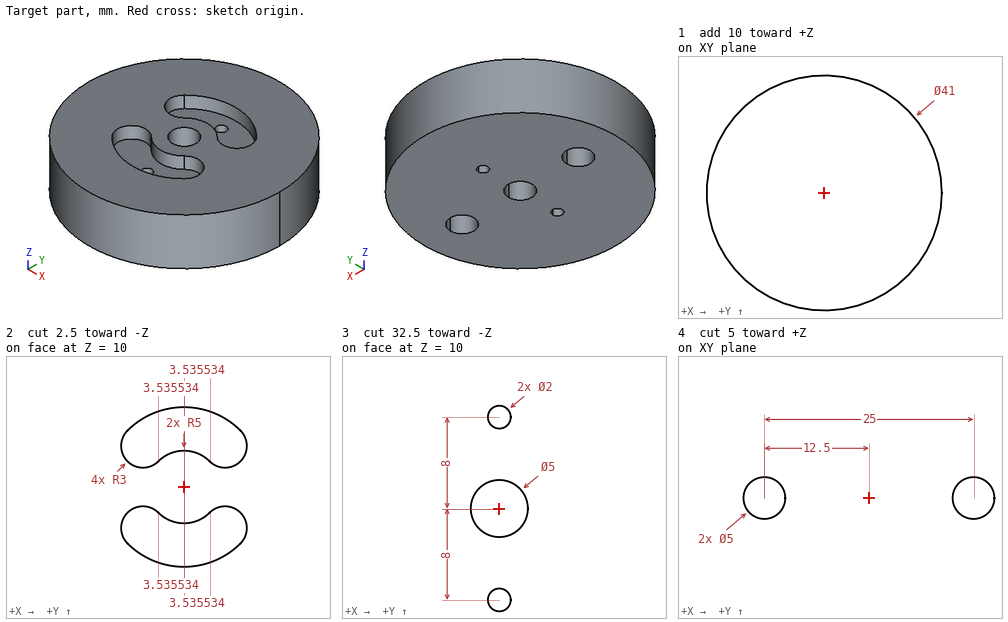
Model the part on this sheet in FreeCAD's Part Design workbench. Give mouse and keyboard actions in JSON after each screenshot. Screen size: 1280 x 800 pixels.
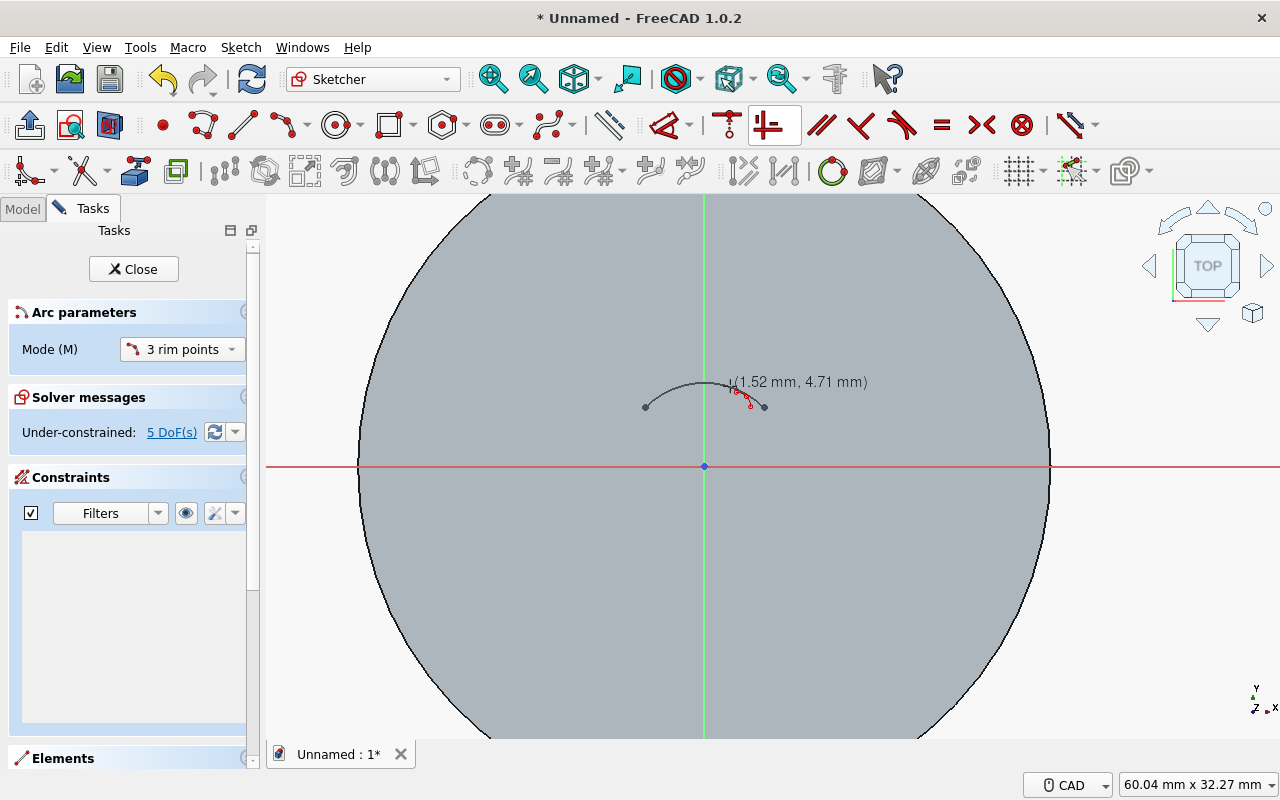
{"action": "left_click", "coordinate": [764, 408]}
{"action": "left_click", "coordinate": [836, 335]}
{"action": "left_click", "coordinate": [836, 407]}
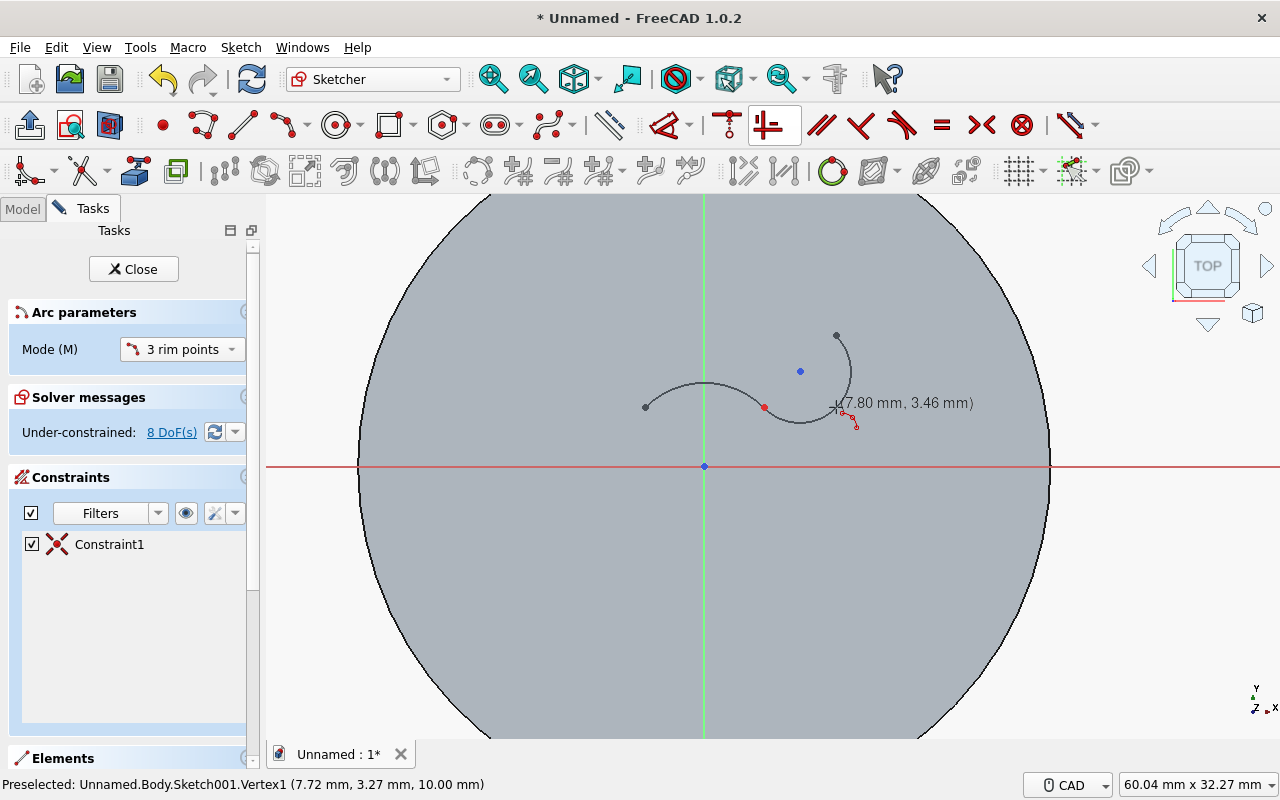
{"action": "left_click", "coordinate": [836, 336]}
{"action": "left_click", "coordinate": [573, 335]}
{"action": "left_click", "coordinate": [733, 283]}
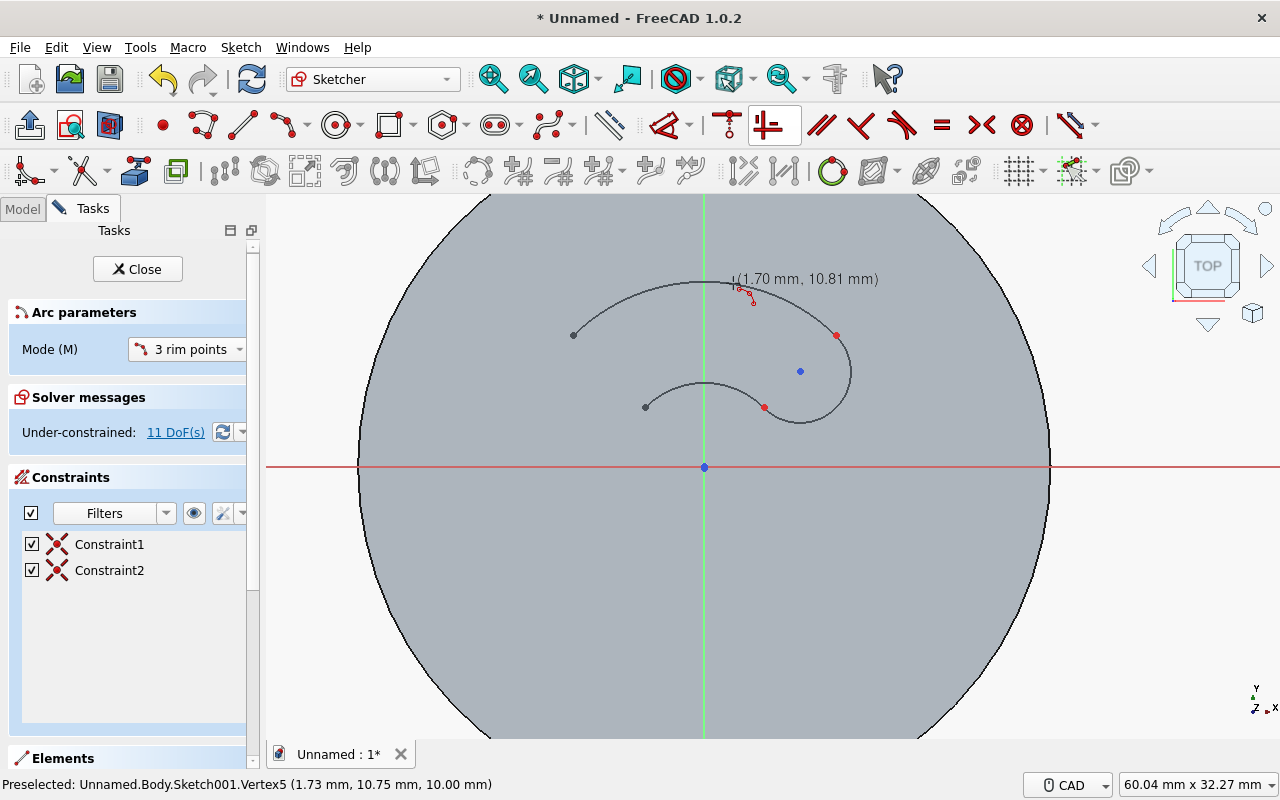
{"action": "left_click", "coordinate": [573, 336]}
{"action": "left_click", "coordinate": [645, 408]}
{"action": "left_click", "coordinate": [573, 407]}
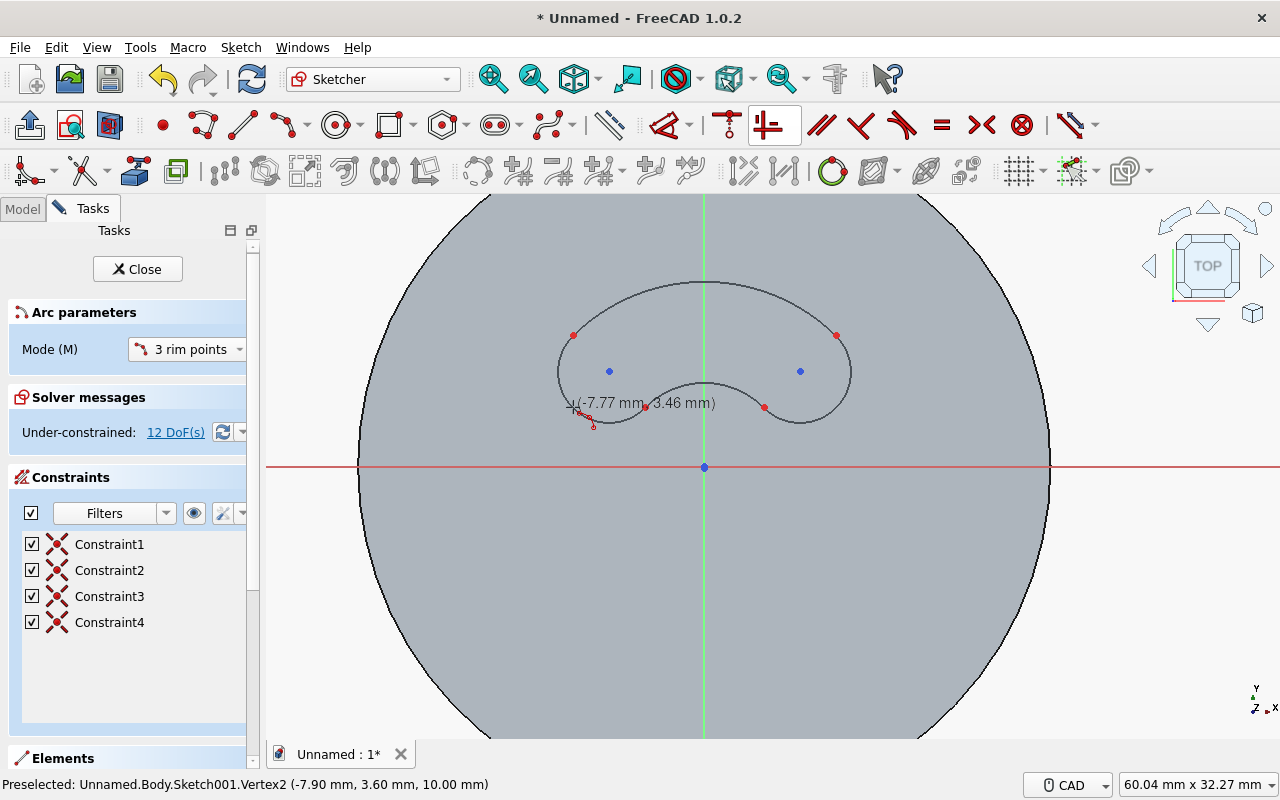
{"action": "left_click", "coordinate": [764, 526]}
{"action": "left_click", "coordinate": [645, 526]}
{"action": "left_click", "coordinate": [678, 547]}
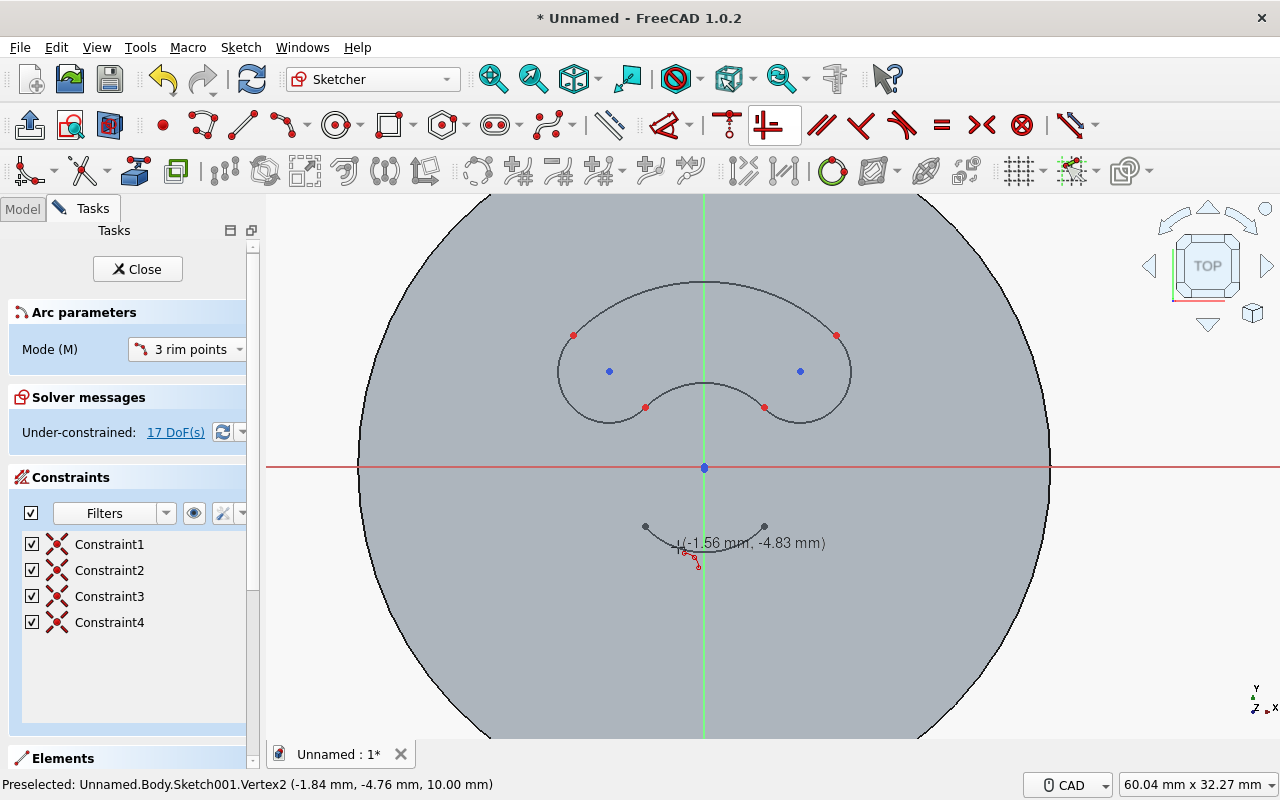
{"action": "left_click", "coordinate": [645, 527]}
{"action": "left_click", "coordinate": [573, 598]}
{"action": "left_click", "coordinate": [573, 526]}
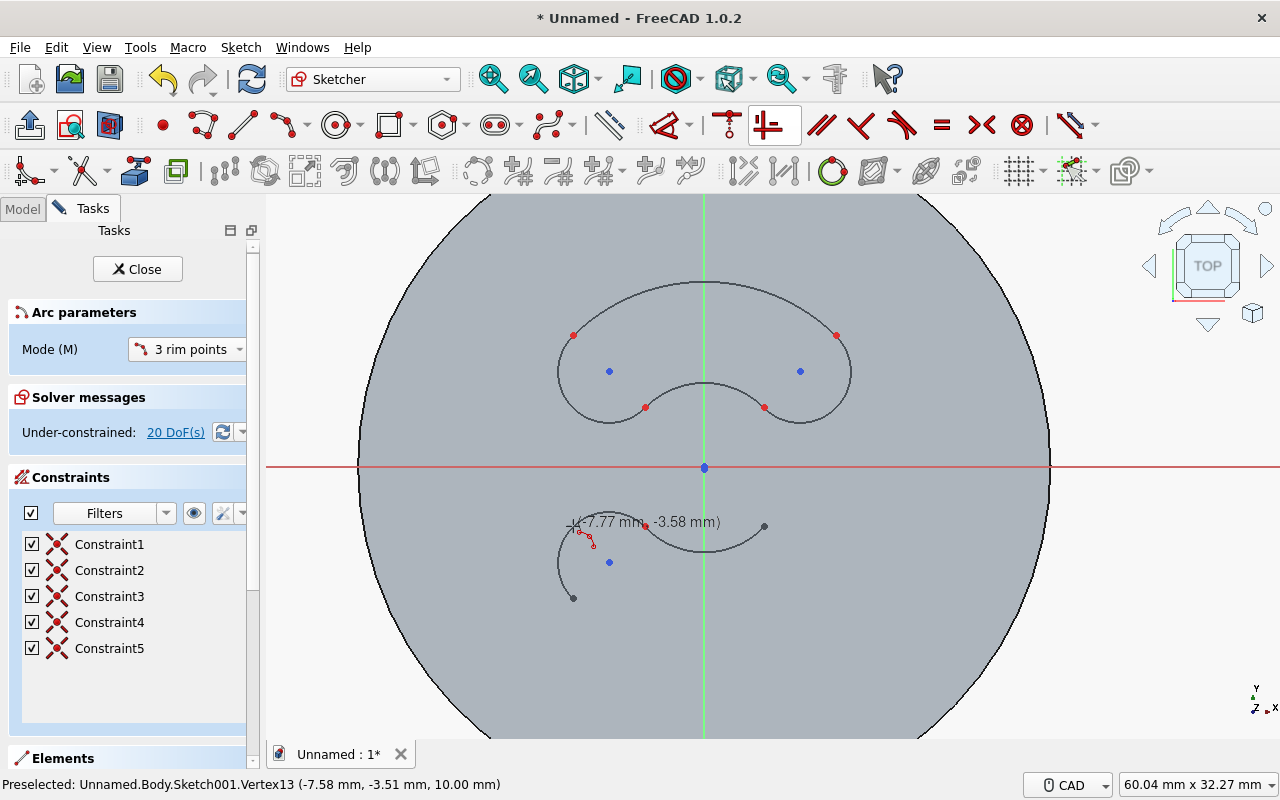
{"action": "left_click", "coordinate": [573, 599]}
{"action": "left_click", "coordinate": [836, 598]}
{"action": "left_click", "coordinate": [675, 650]}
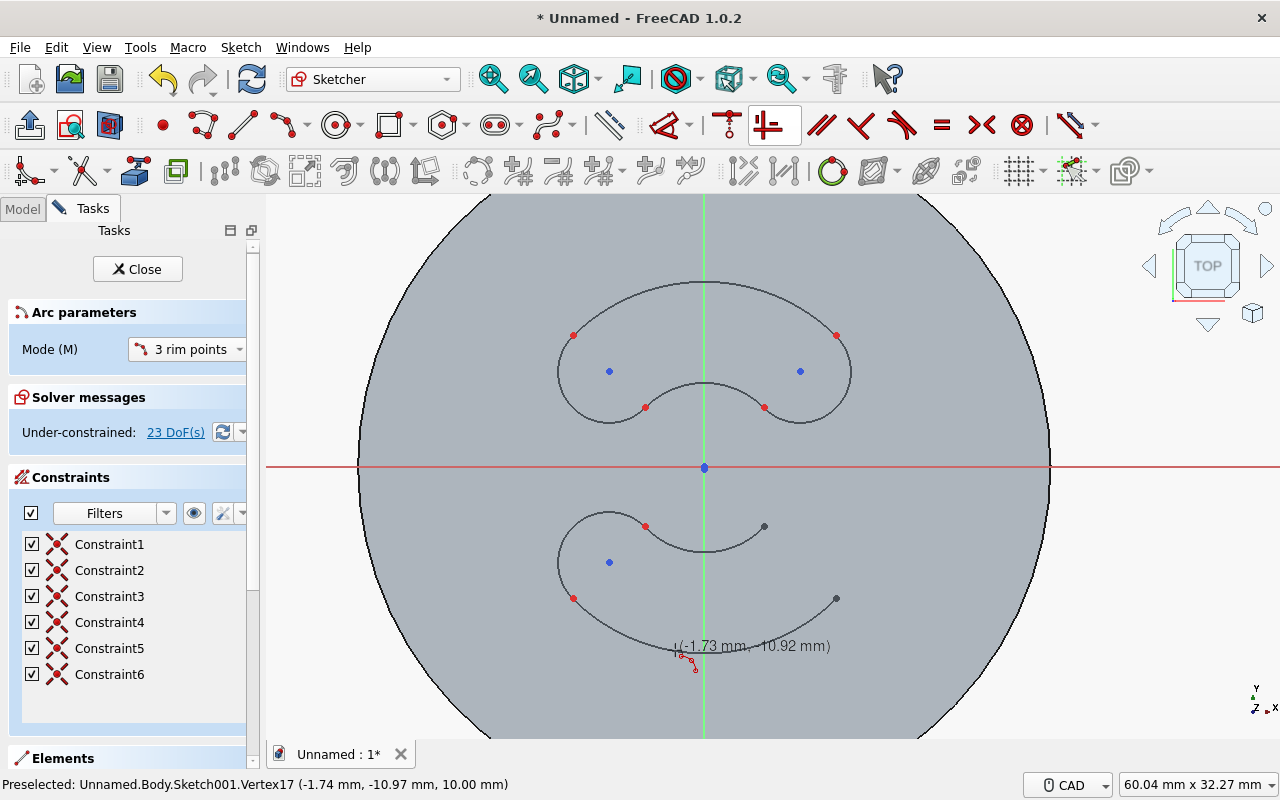
{"action": "left_click", "coordinate": [836, 599]}
{"action": "left_click", "coordinate": [764, 527]}
{"action": "left_click", "coordinate": [836, 526]}
{"action": "key", "text": "Escape"}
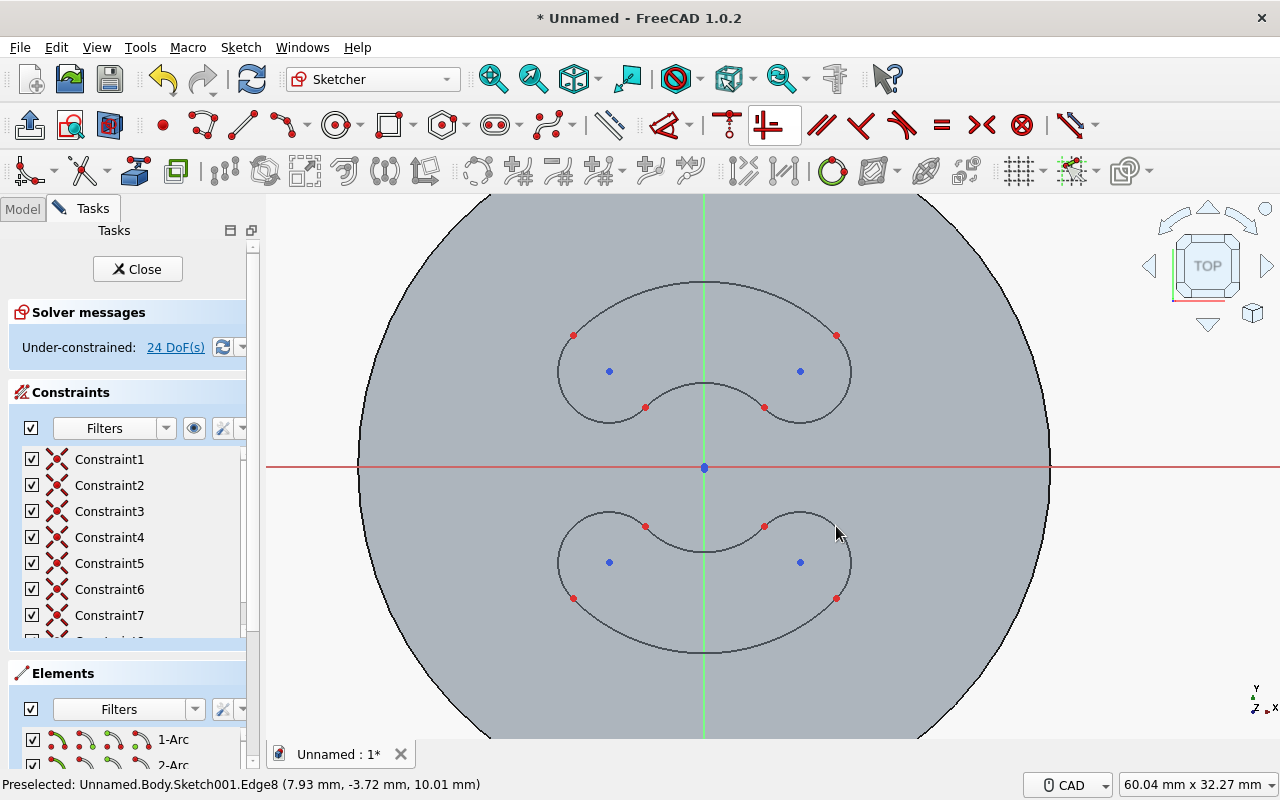
{"action": "left_click", "coordinate": [731, 387]}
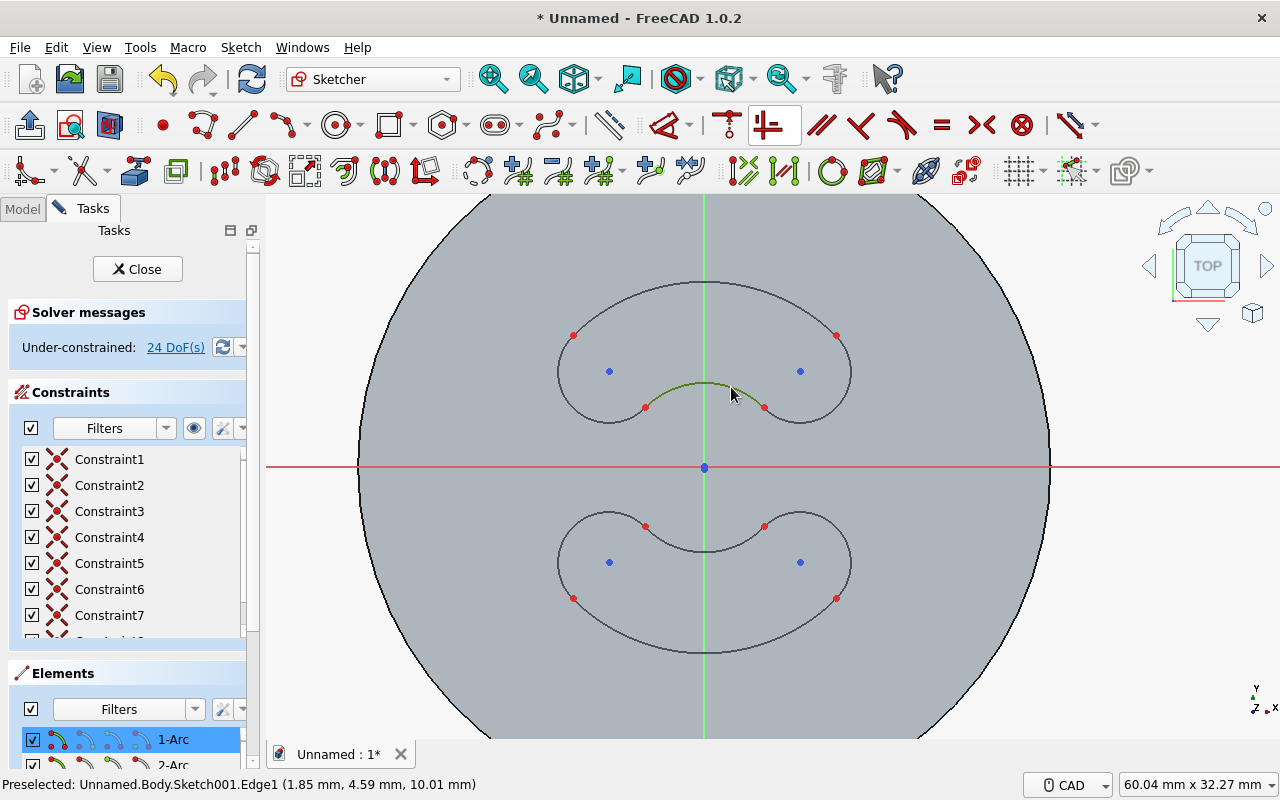
{"action": "left_click", "coordinate": [808, 422]}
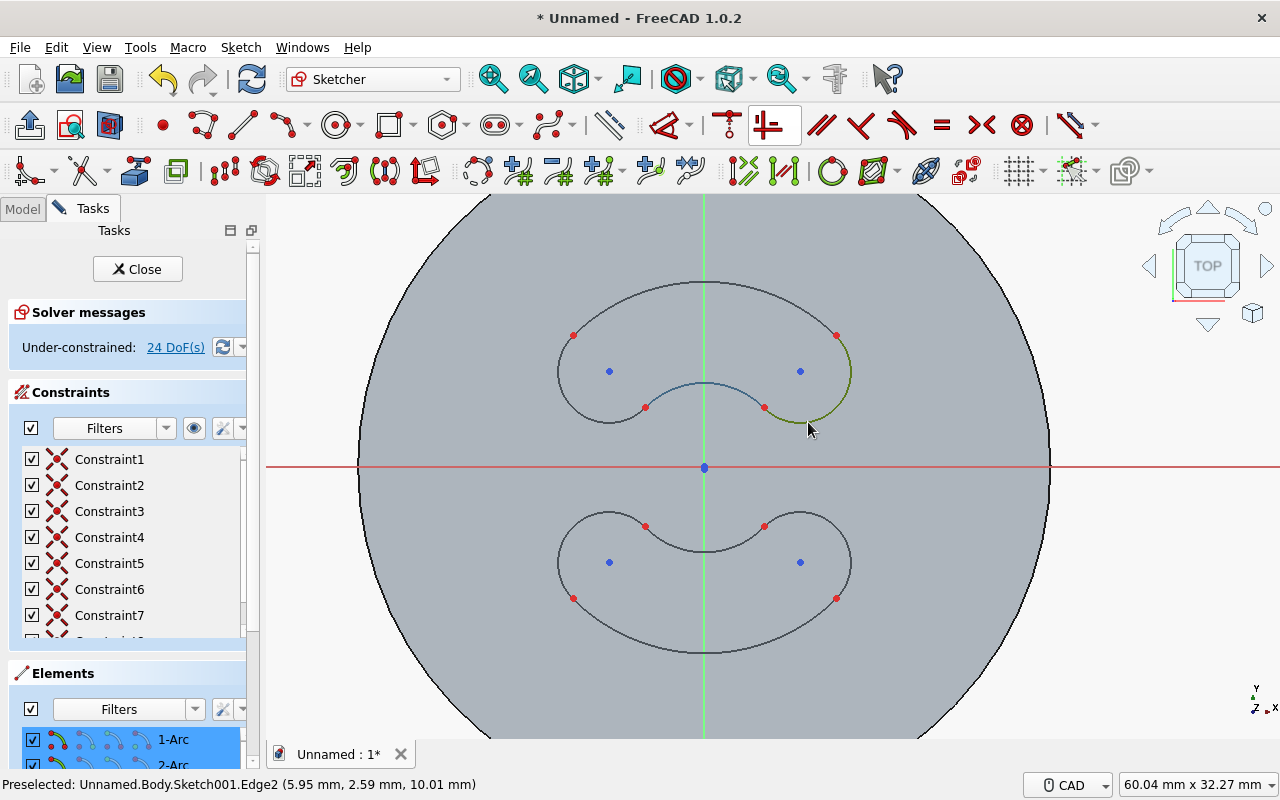
{"action": "key", "text": "t"}